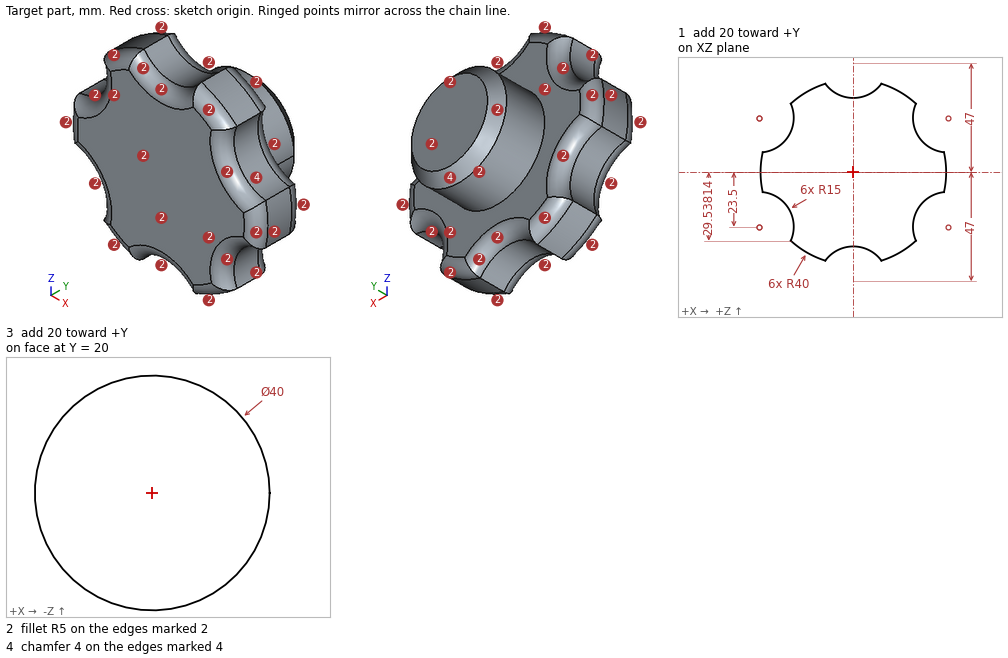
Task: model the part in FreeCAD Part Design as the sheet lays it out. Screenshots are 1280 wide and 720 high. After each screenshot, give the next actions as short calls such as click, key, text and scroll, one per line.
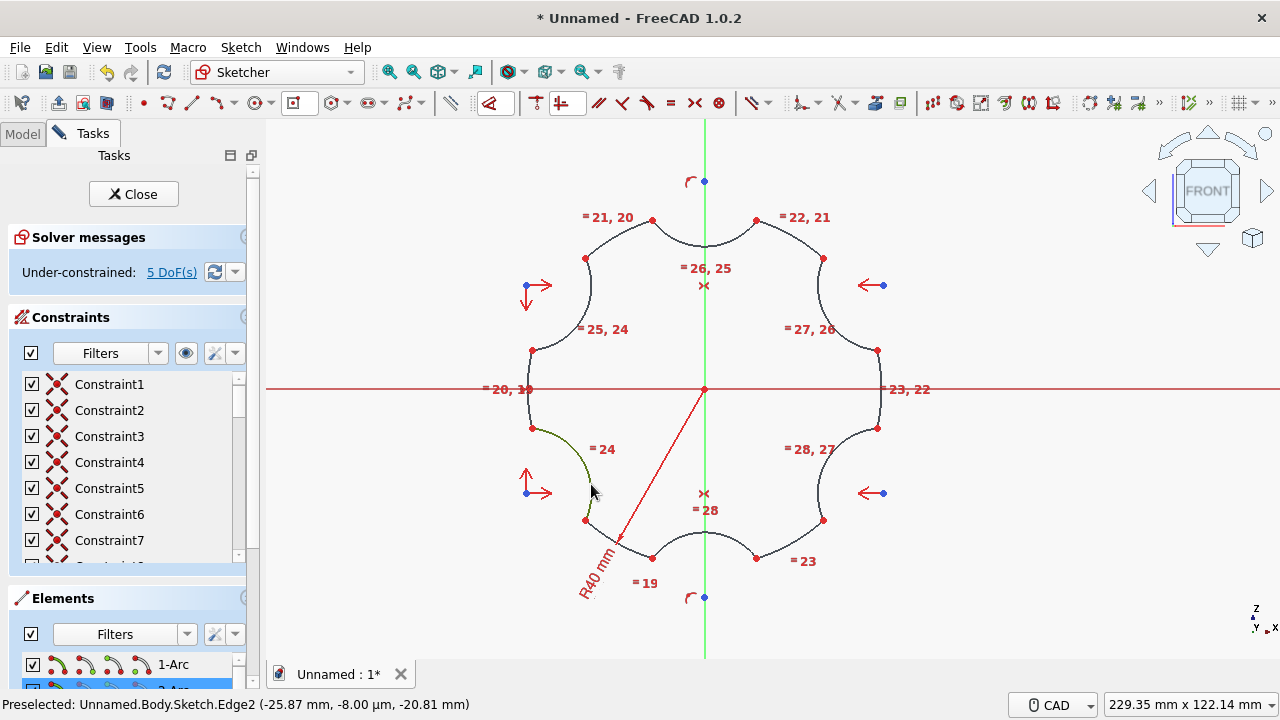
key(k)
key(r)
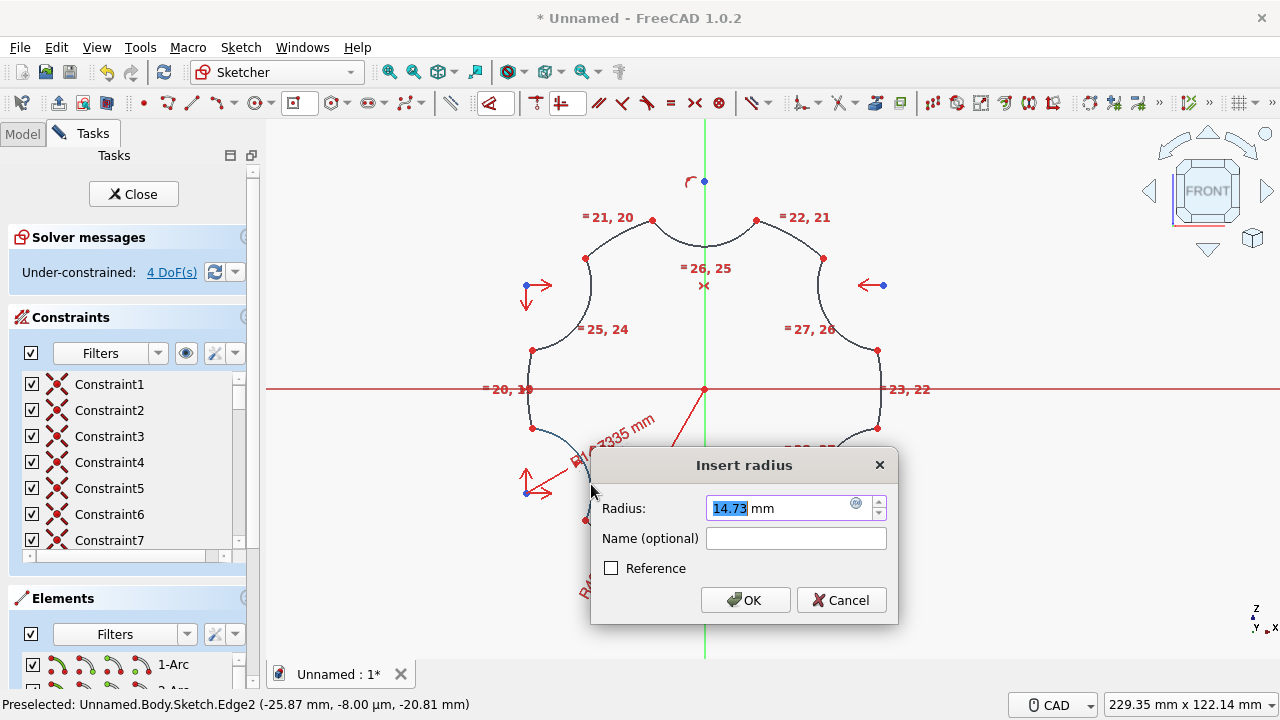
text(15)
key(Return)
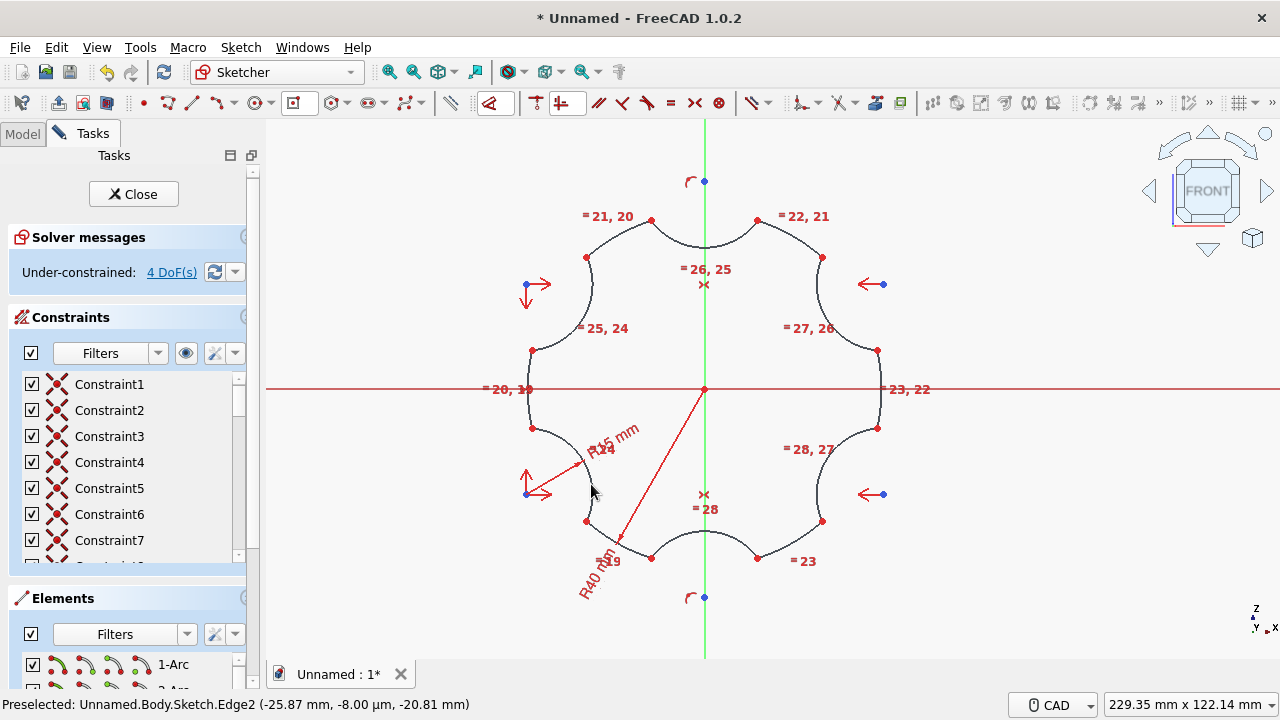
click(705, 181)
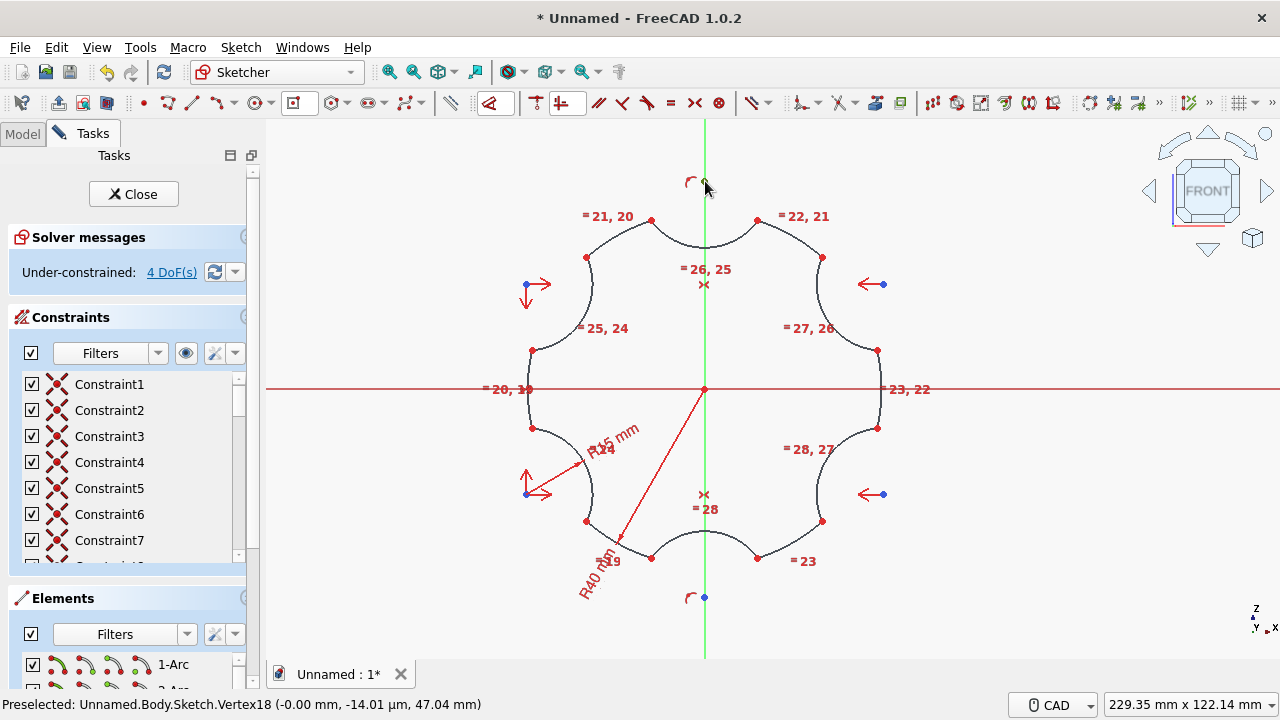
key(i)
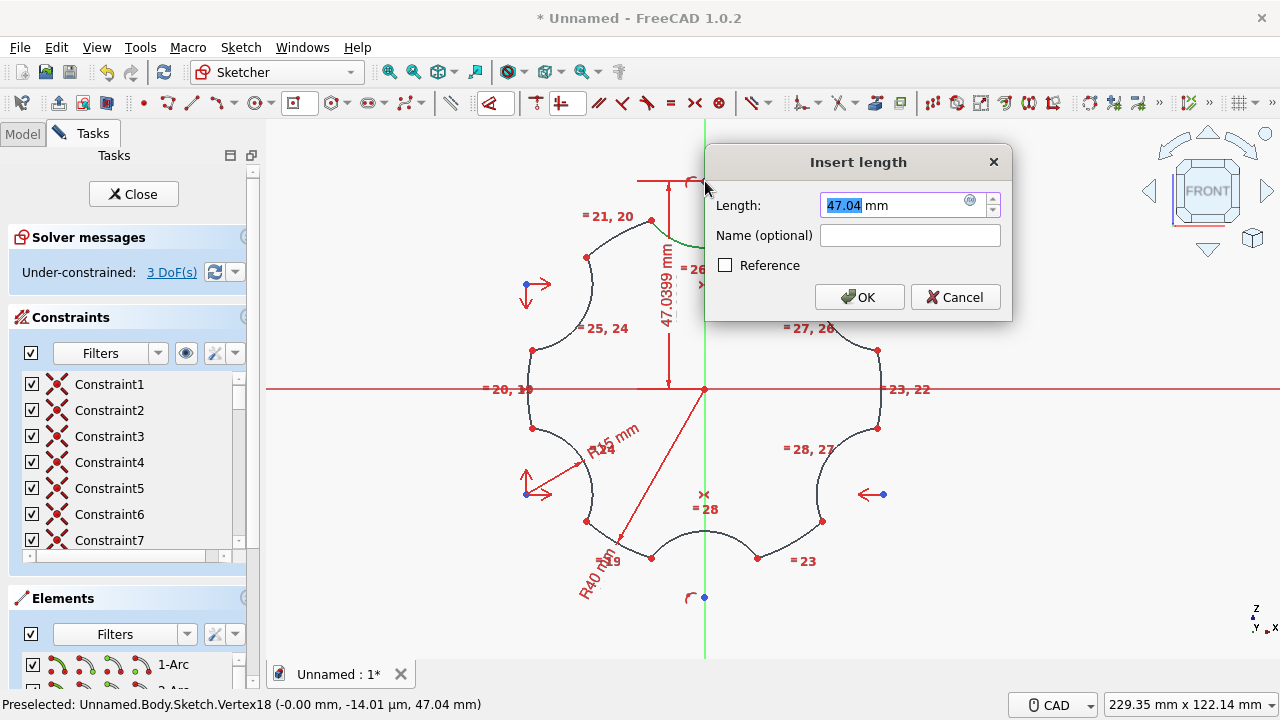
text(47)
key(Return)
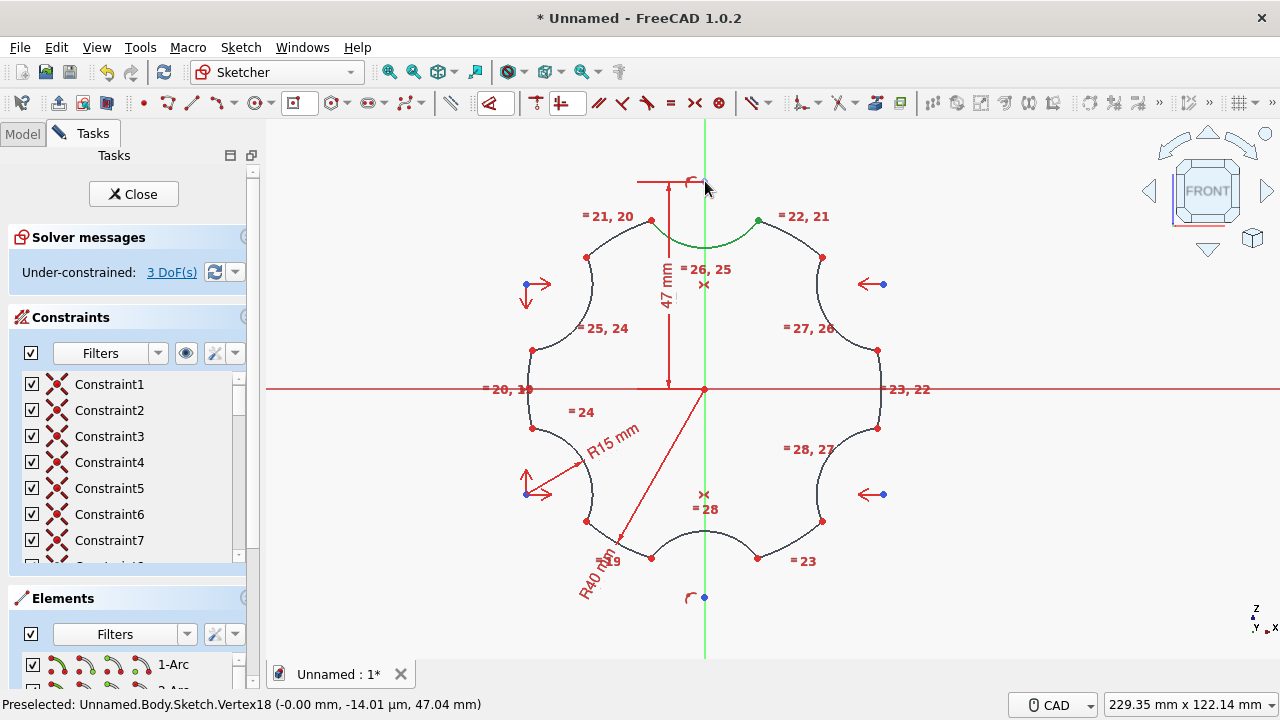
click(705, 598)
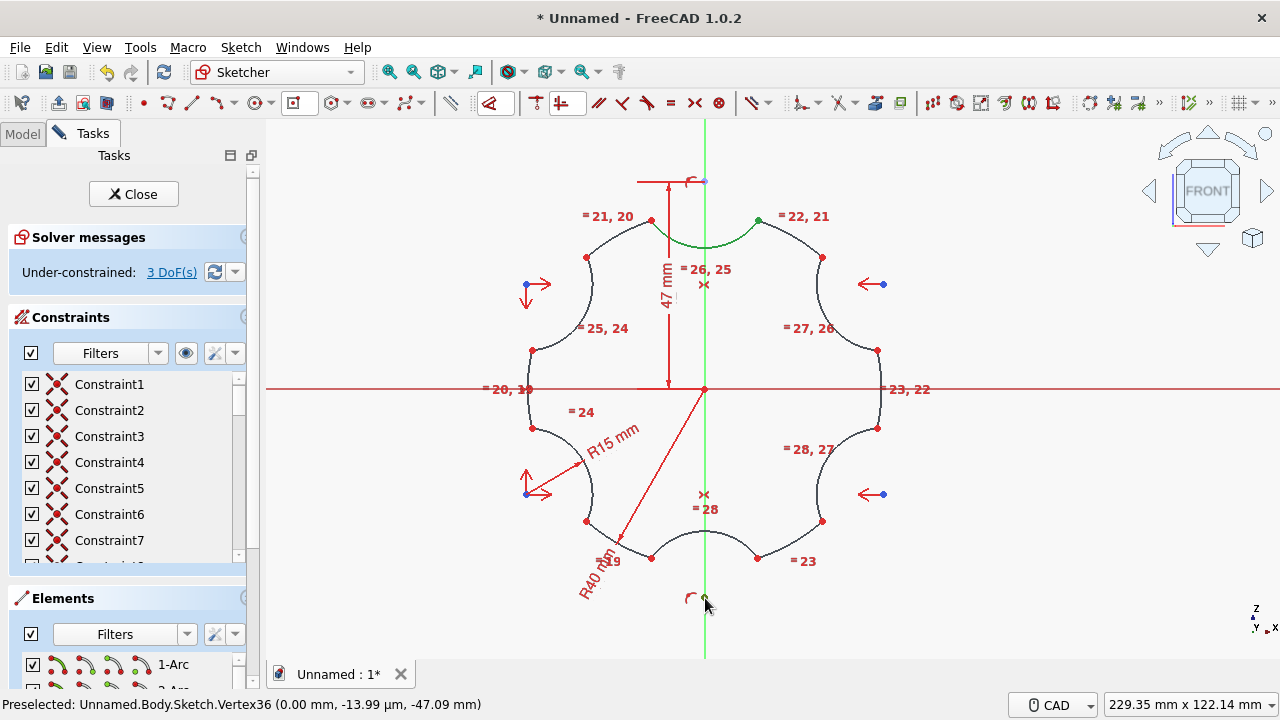
click(508, 104)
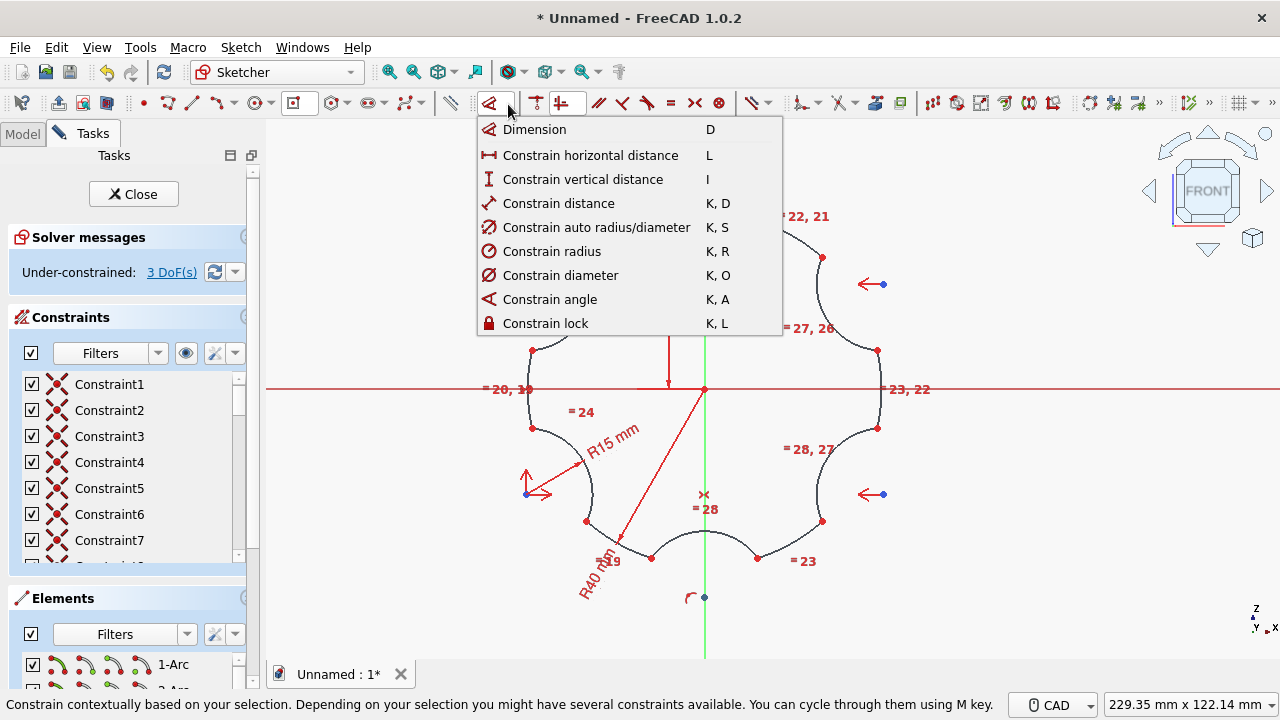
click(630, 179)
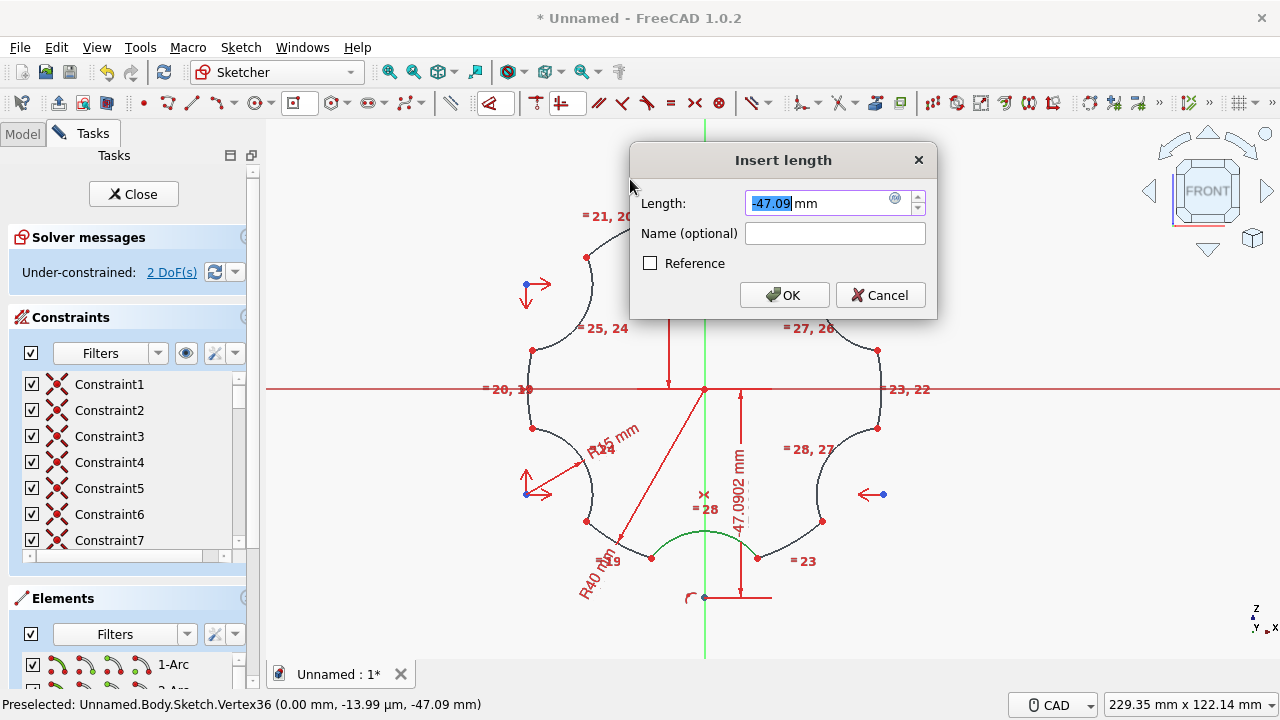
text(-47)
key(Return)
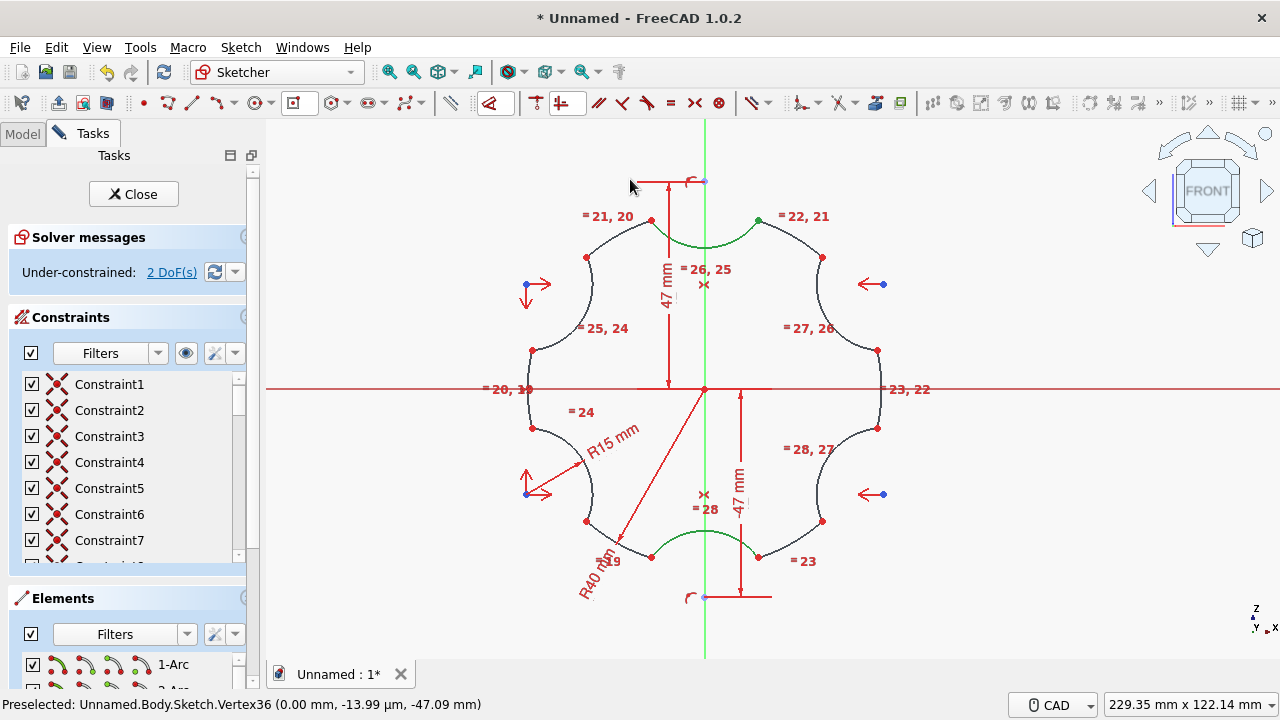
click(526, 495)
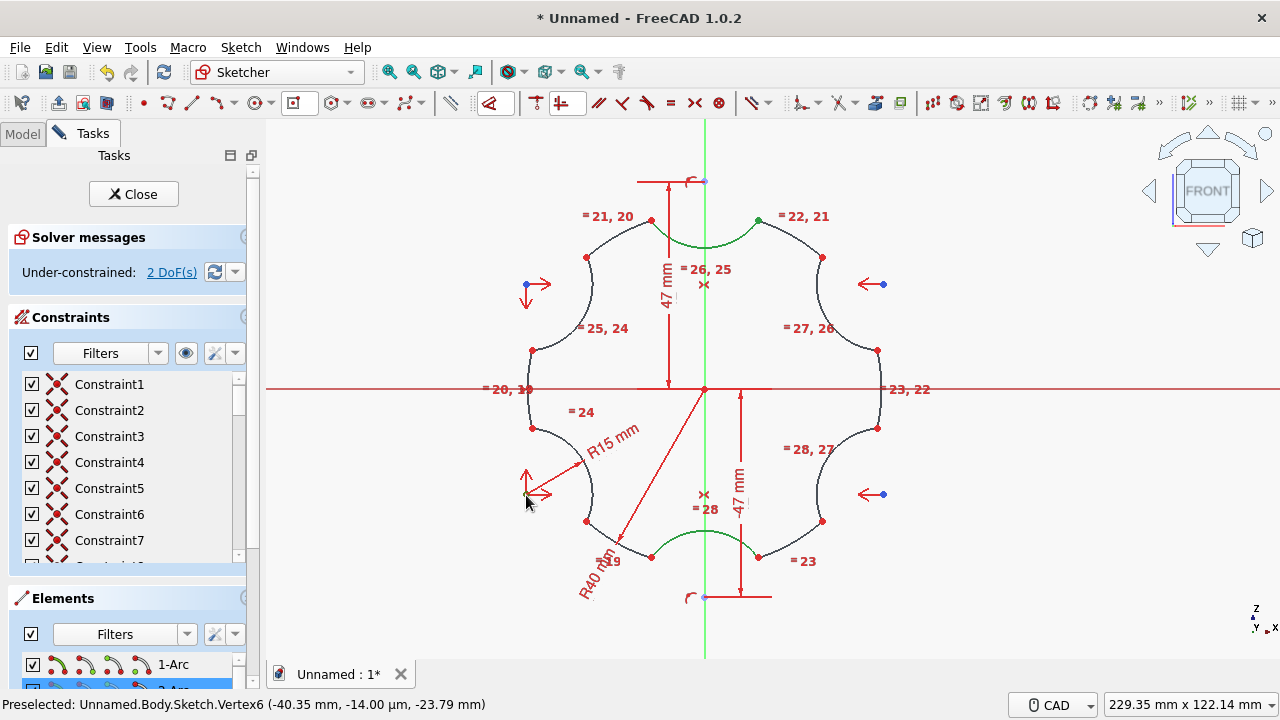
click(508, 104)